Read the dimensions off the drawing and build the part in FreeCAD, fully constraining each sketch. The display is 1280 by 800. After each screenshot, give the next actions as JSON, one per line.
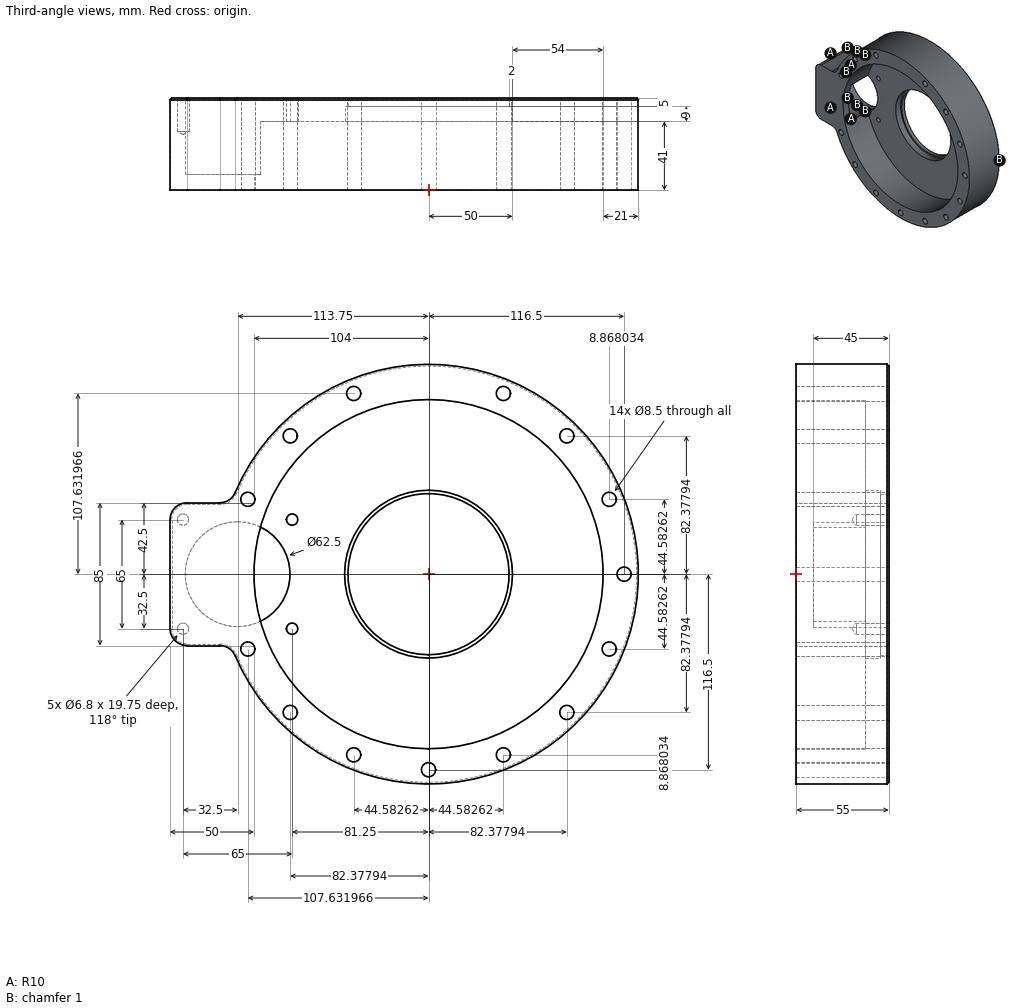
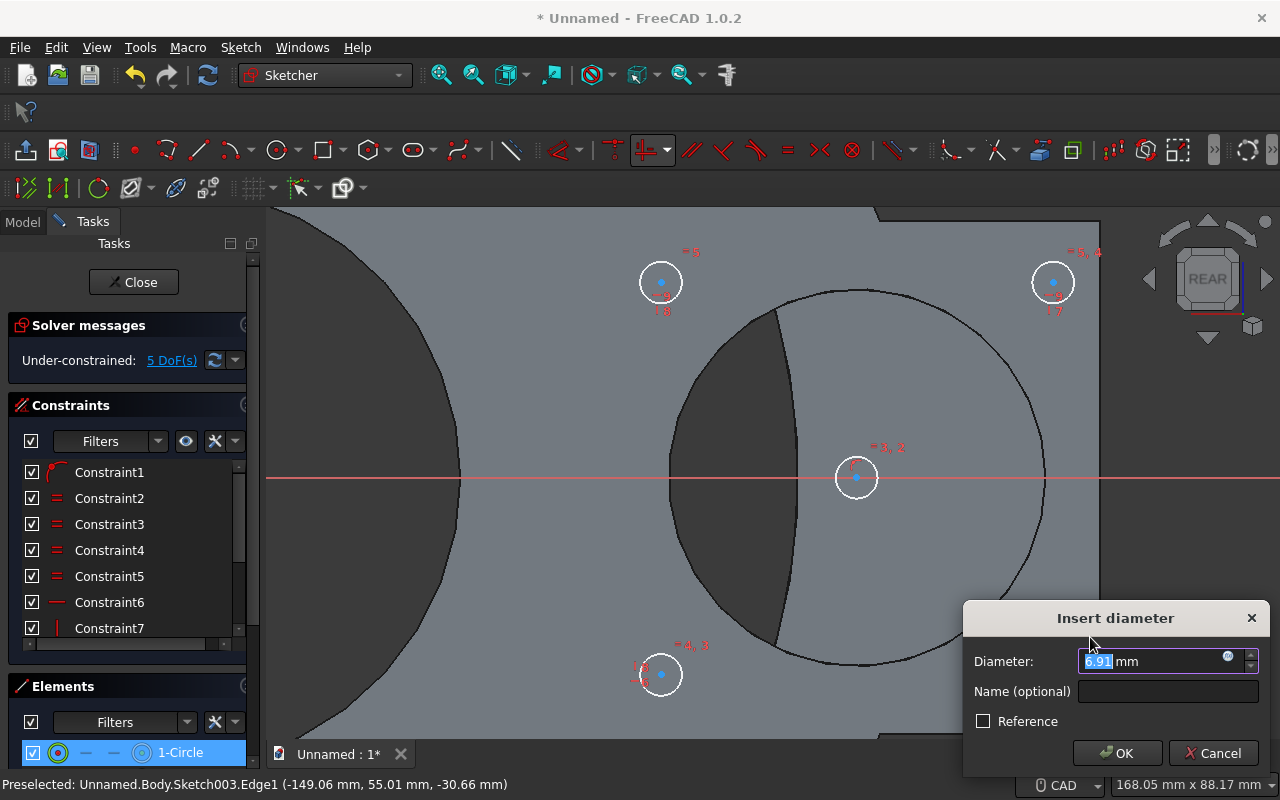
{"action": "type", "text": "6.8"}
{"action": "key", "text": "Return"}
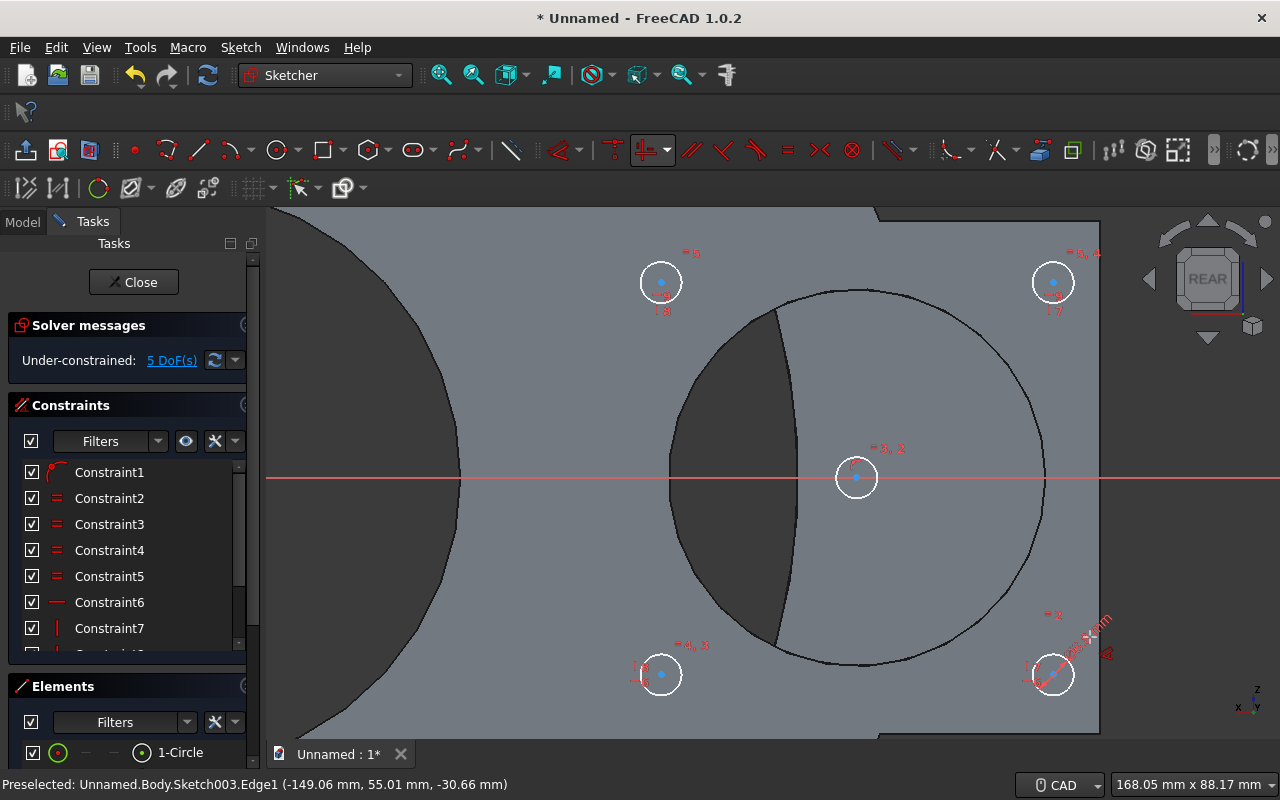
{"action": "left_click", "coordinate": [1053, 675]}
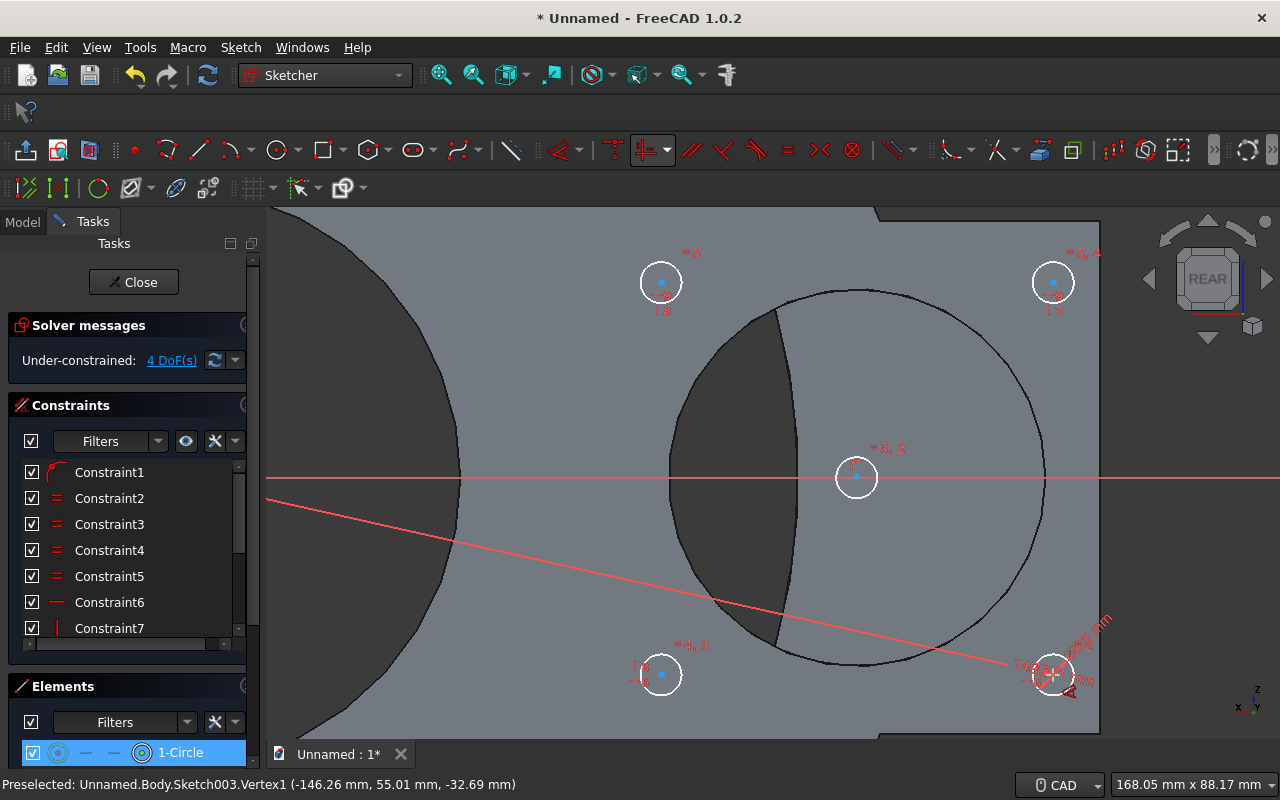
{"action": "left_click", "coordinate": [661, 675]}
{"action": "left_click", "coordinate": [857, 709]}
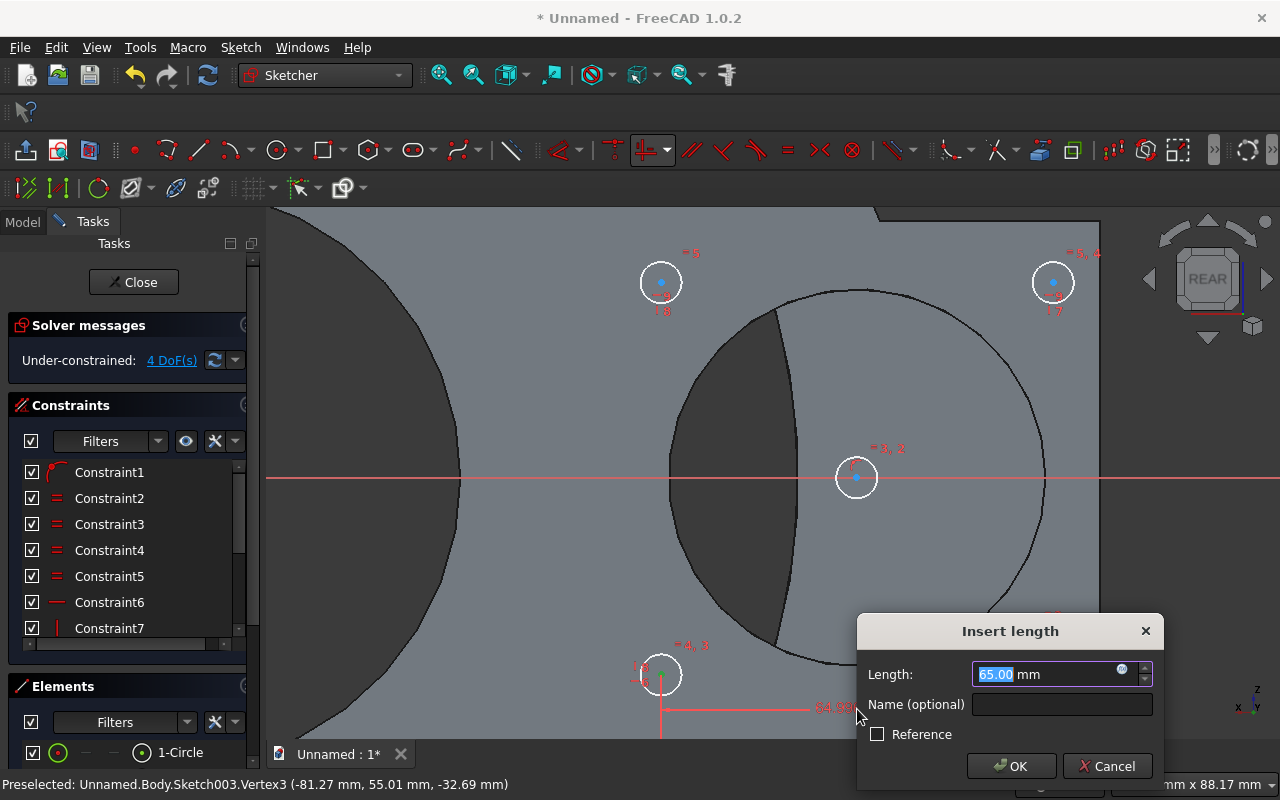
{"action": "type", "text": "65"}
{"action": "key", "text": "Return"}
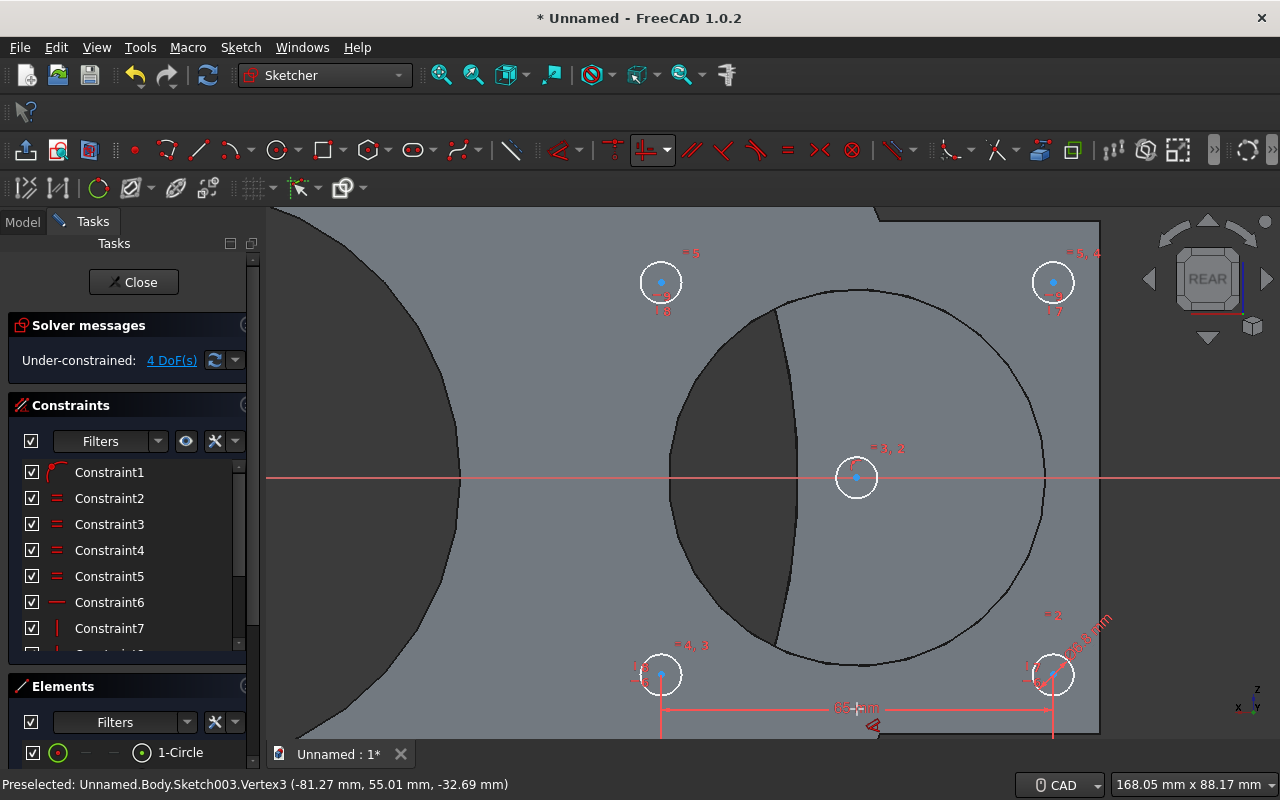
{"action": "left_click", "coordinate": [1053, 675]}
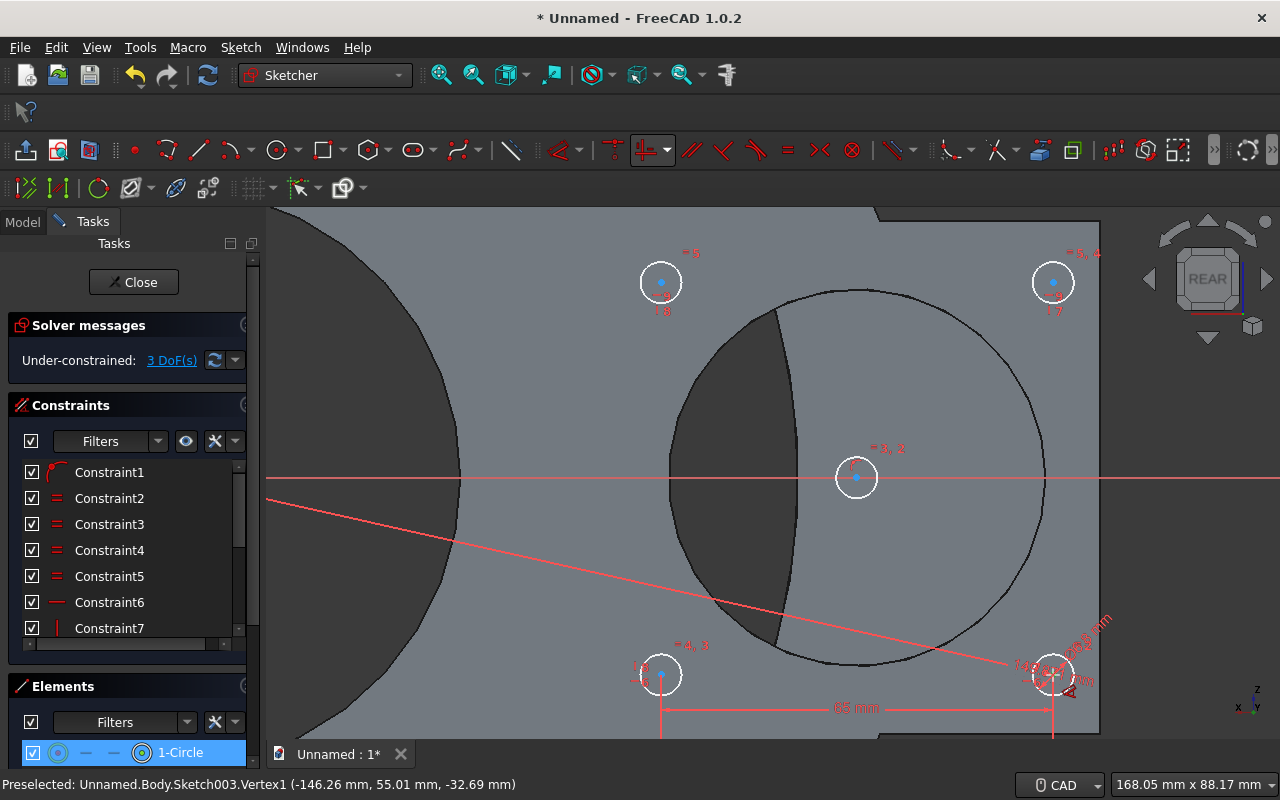
{"action": "left_click", "coordinate": [1053, 283]}
{"action": "left_click", "coordinate": [1087, 389]}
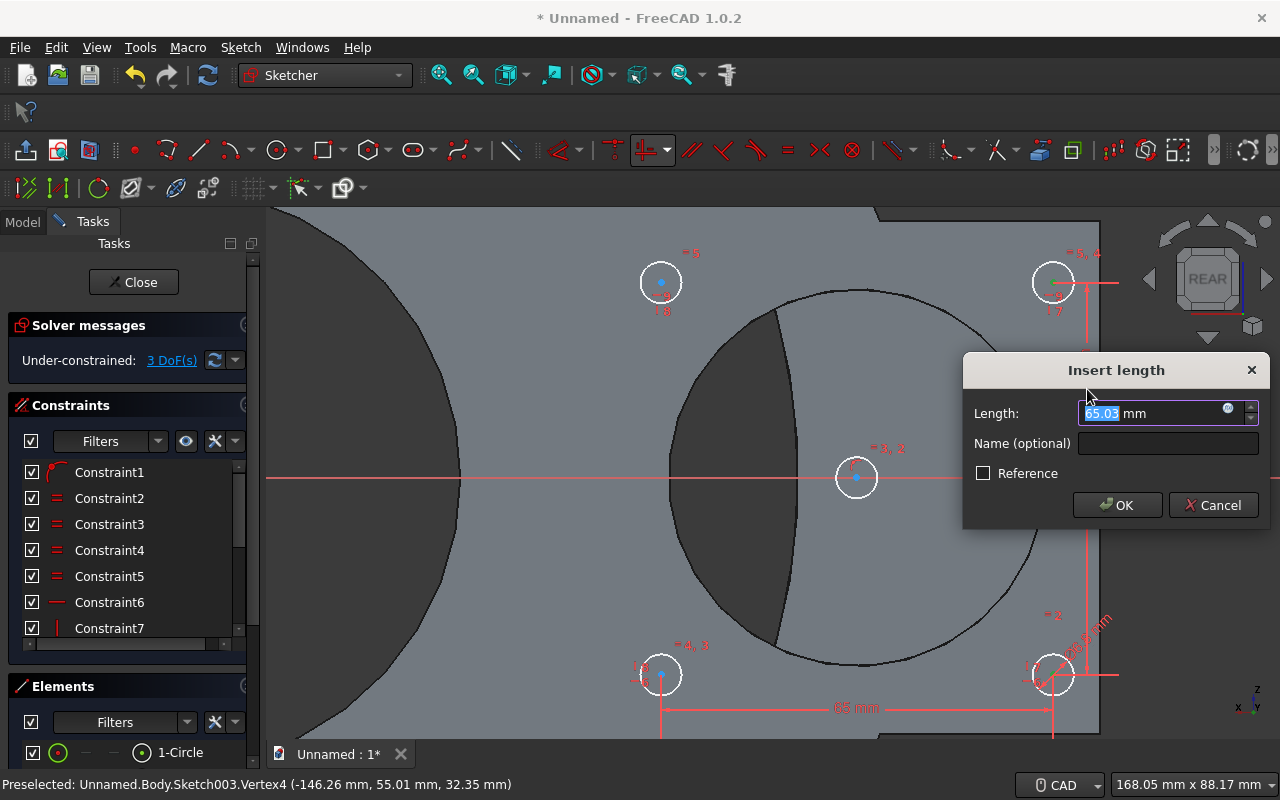
{"action": "type", "text": "65"}
{"action": "key", "text": "Return"}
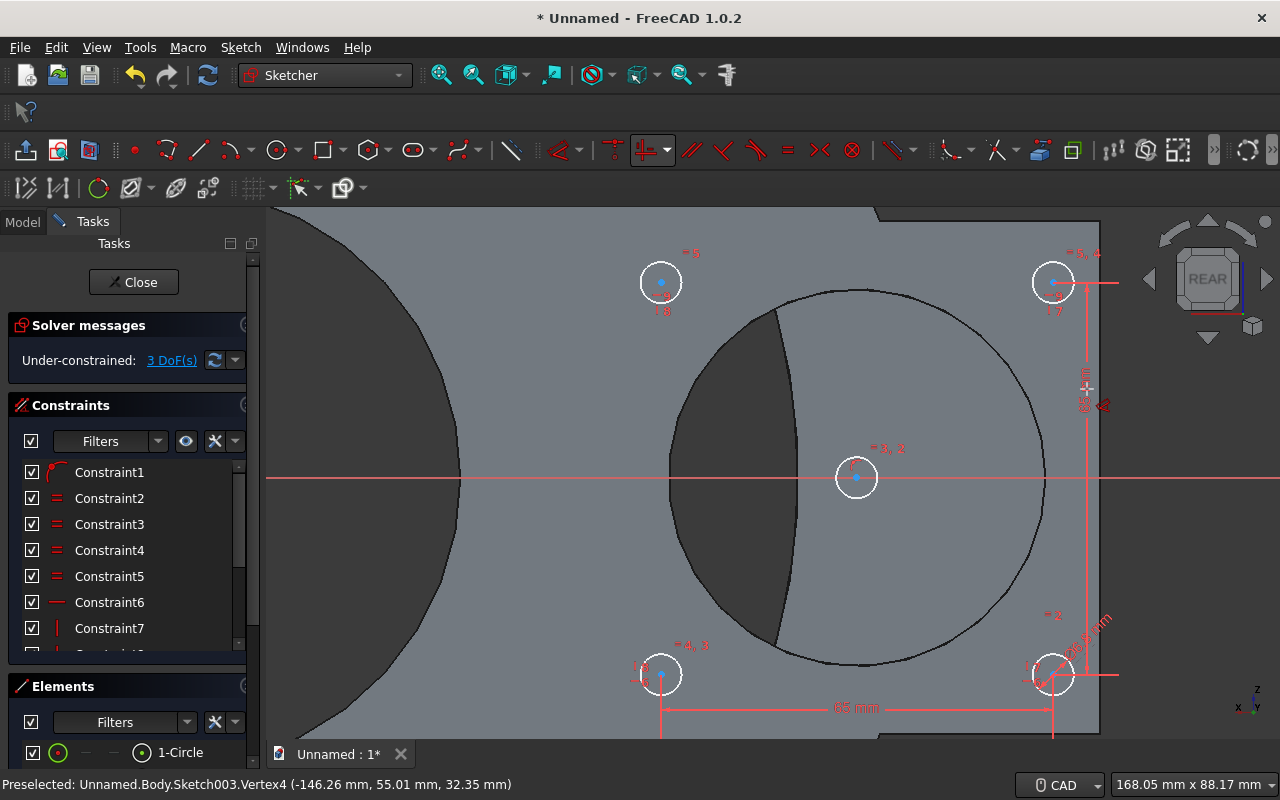
{"action": "left_click", "coordinate": [1053, 675]}
{"action": "left_click", "coordinate": [1087, 576]}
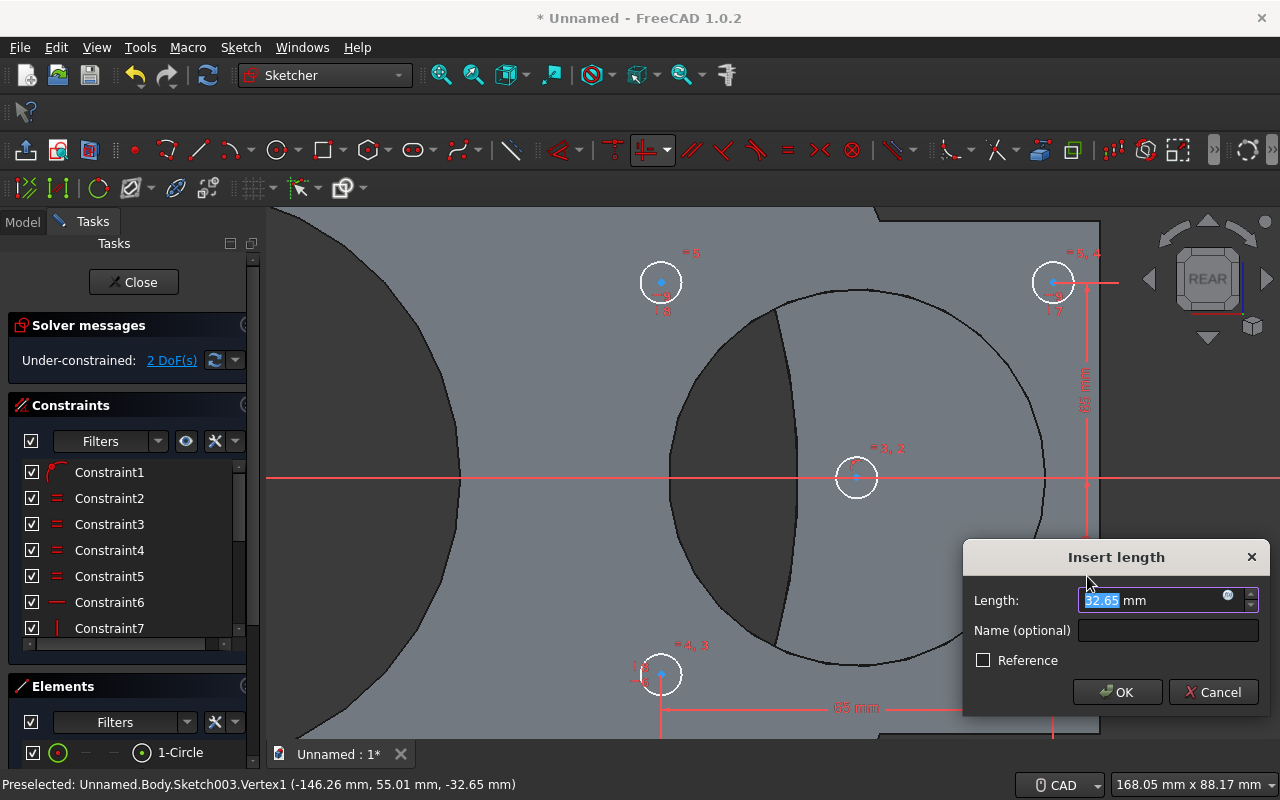
{"action": "type", "text": "32.5"}
{"action": "key", "text": "Return"}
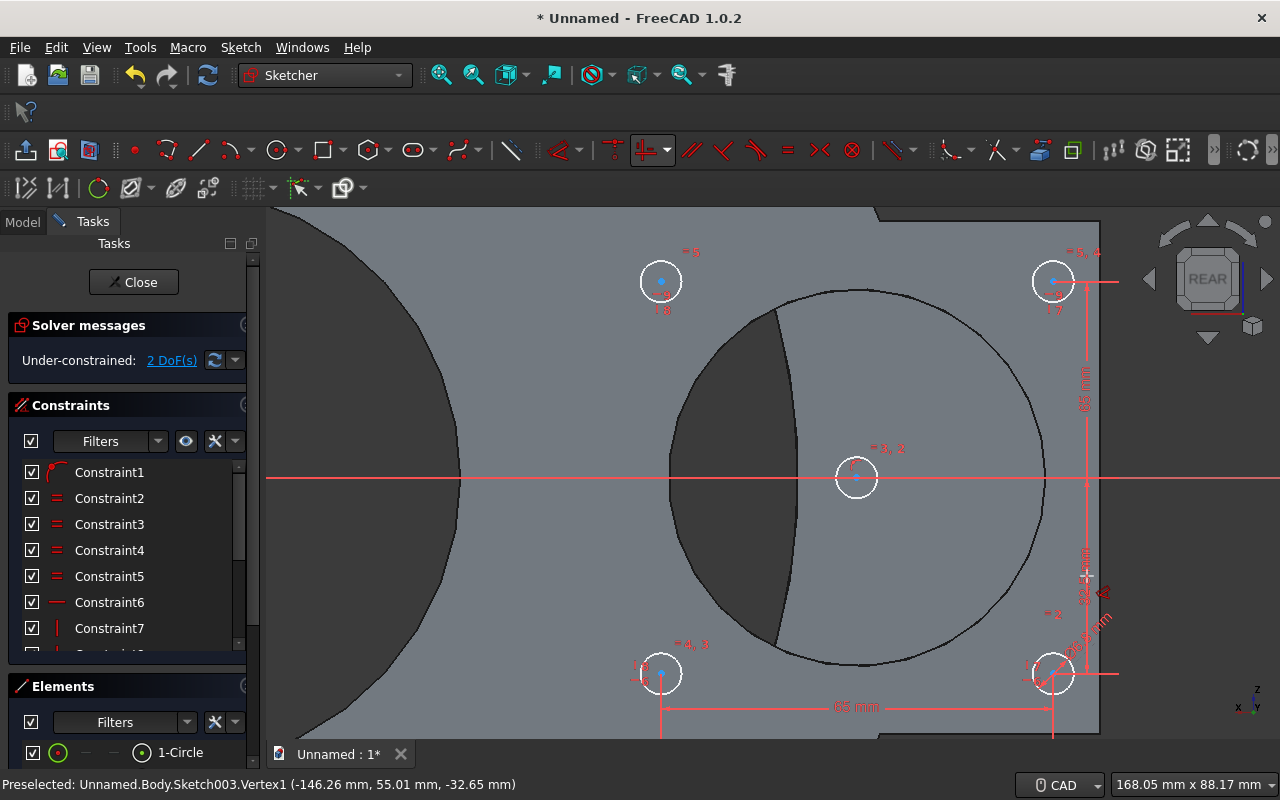
{"action": "left_click", "coordinate": [661, 674]}
{"action": "left_click", "coordinate": [478, 708]}